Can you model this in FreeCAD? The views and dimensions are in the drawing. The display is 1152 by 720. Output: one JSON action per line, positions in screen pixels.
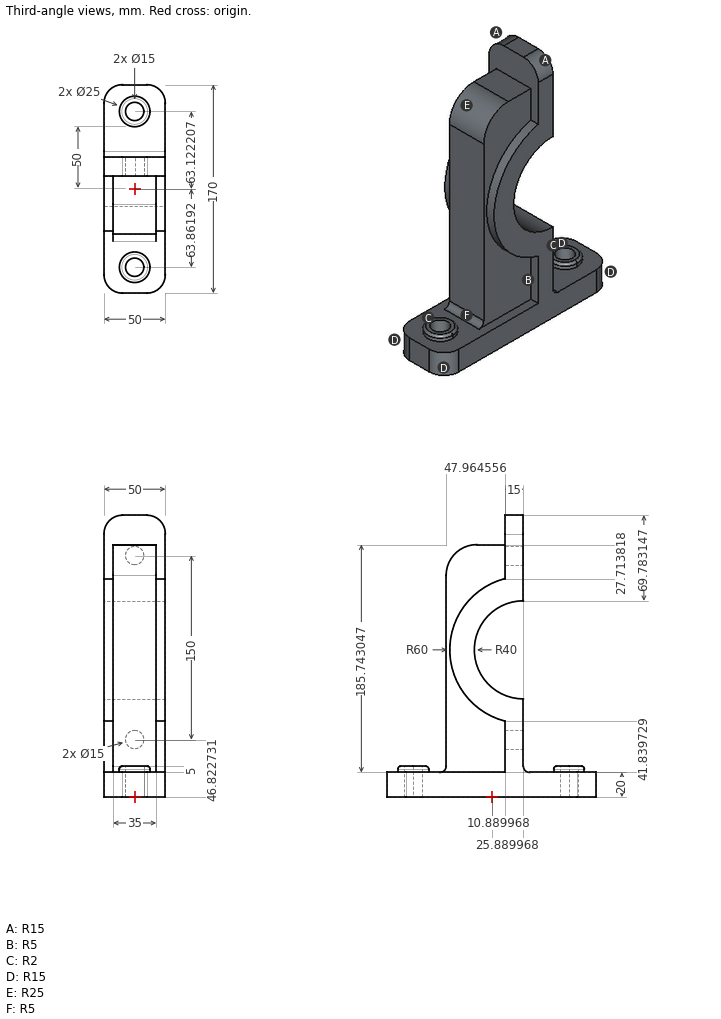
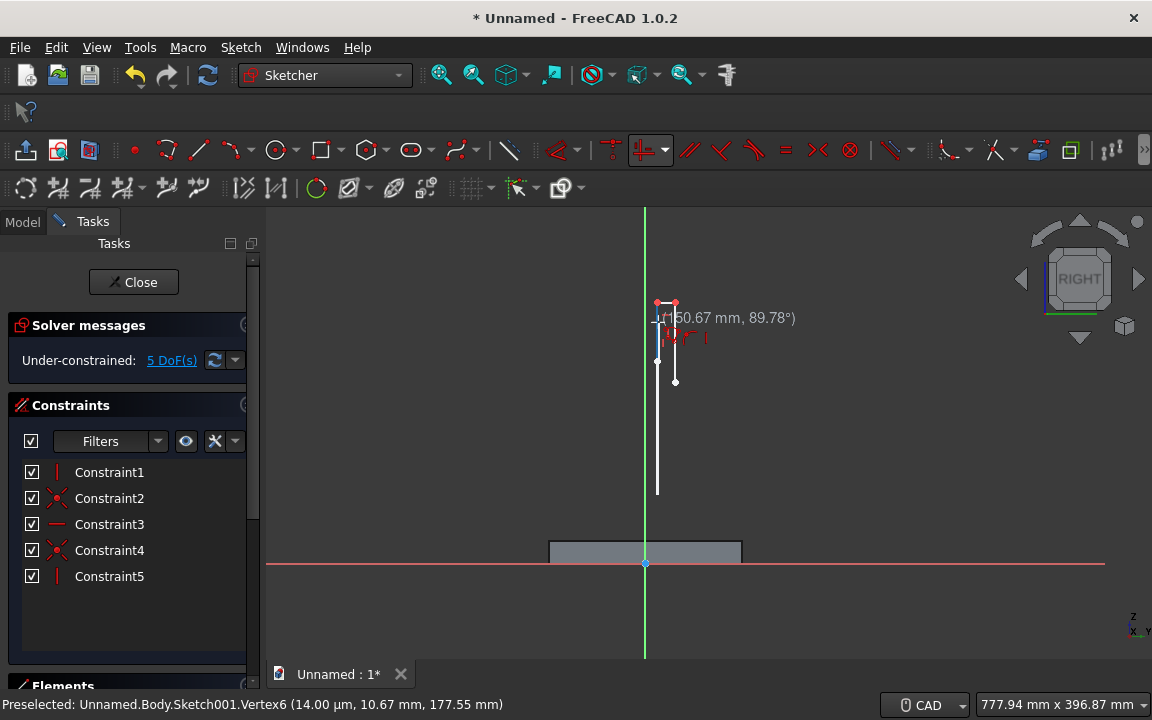
{"action": "scroll", "coordinate": [658, 541], "scroll_direction": "up", "scroll_amount": 2}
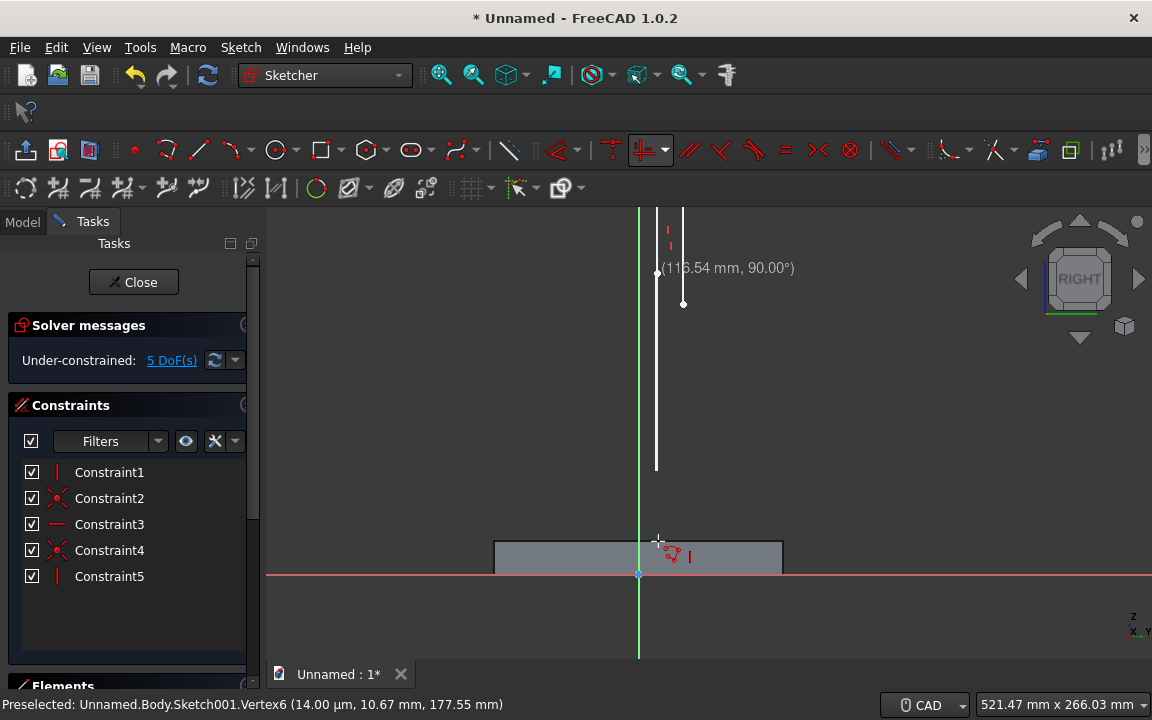
{"action": "left_click", "coordinate": [657, 541]}
{"action": "left_click", "coordinate": [683, 541]}
{"action": "left_click", "coordinate": [683, 439]}
{"action": "right_click", "coordinate": [683, 439]}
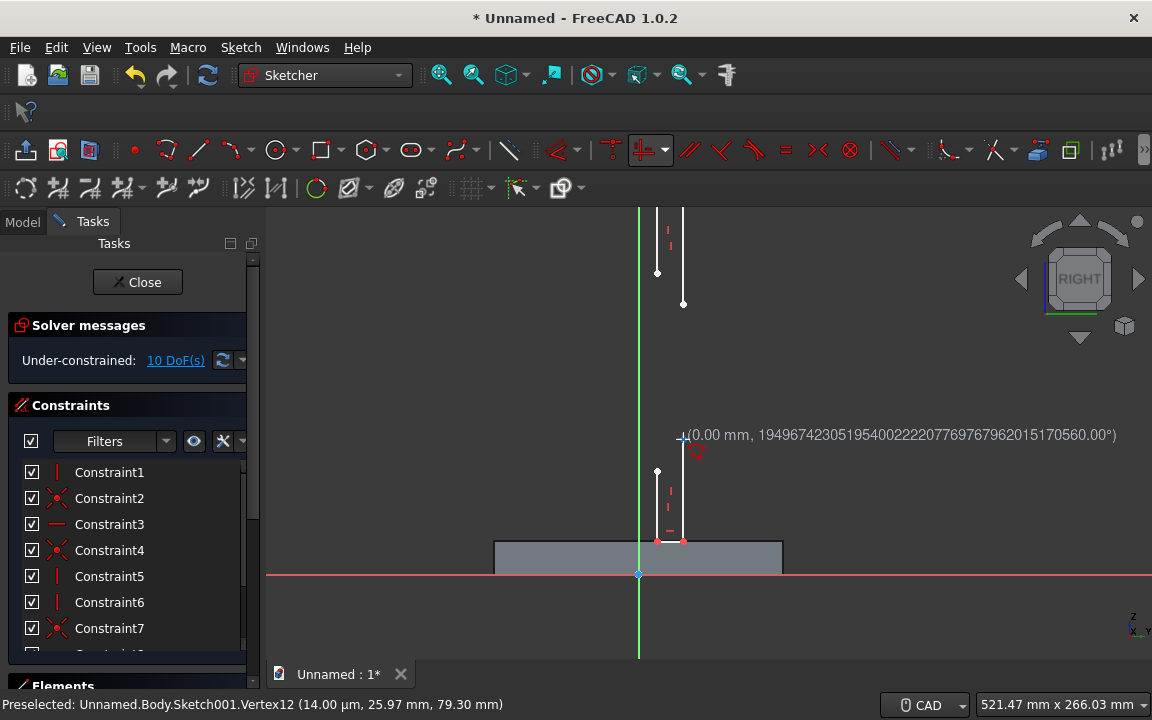
{"action": "key", "text": "g 3 a"}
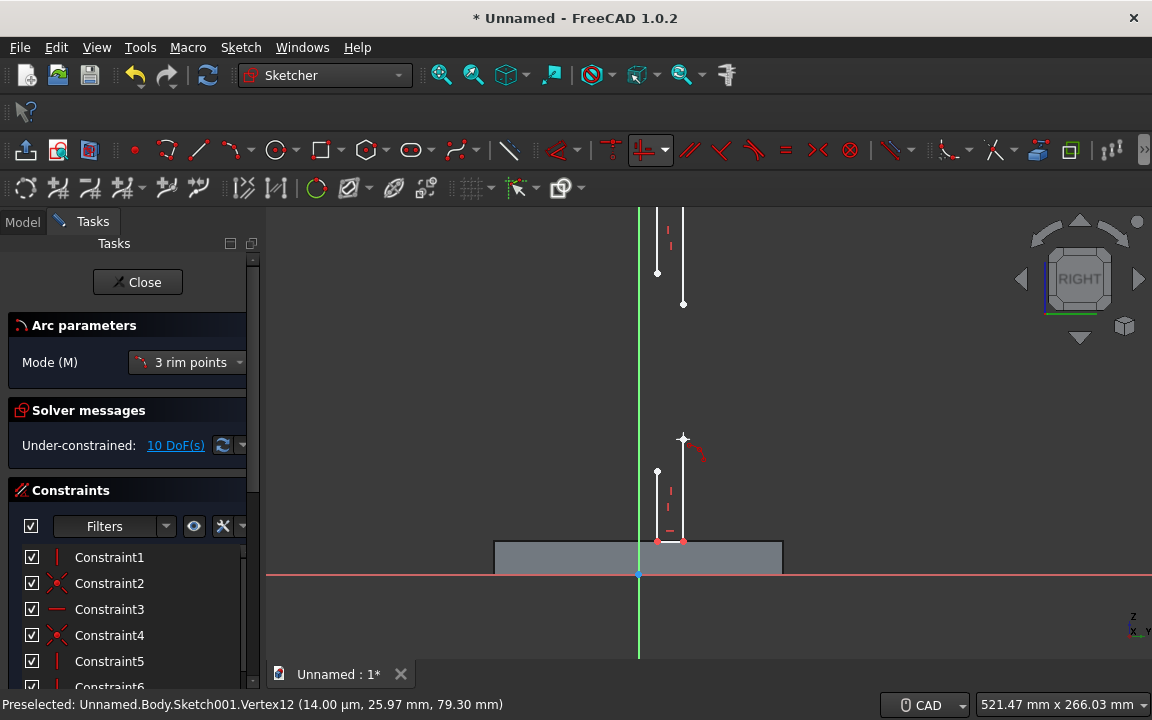
{"action": "left_click", "coordinate": [657, 273]}
{"action": "left_click", "coordinate": [657, 471]}
{"action": "left_click", "coordinate": [581, 371]}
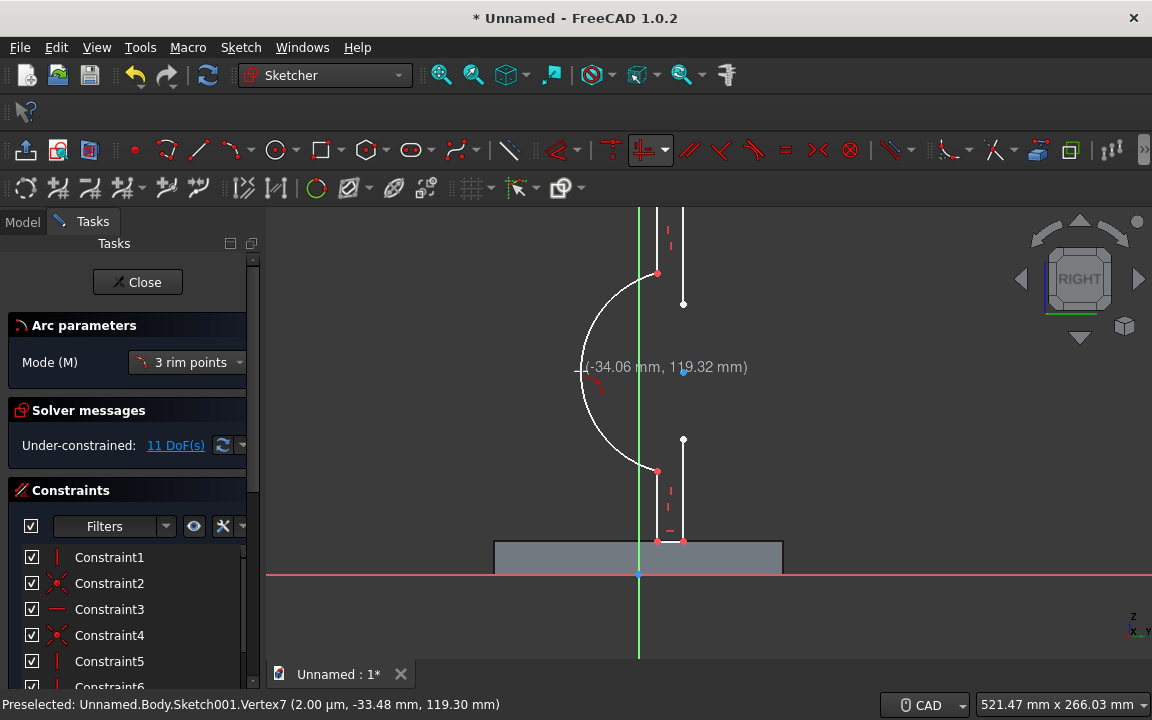
{"action": "left_click", "coordinate": [683, 440]}
{"action": "left_click", "coordinate": [683, 305]}
{"action": "left_click", "coordinate": [615, 371]}
{"action": "key", "text": "Escape"}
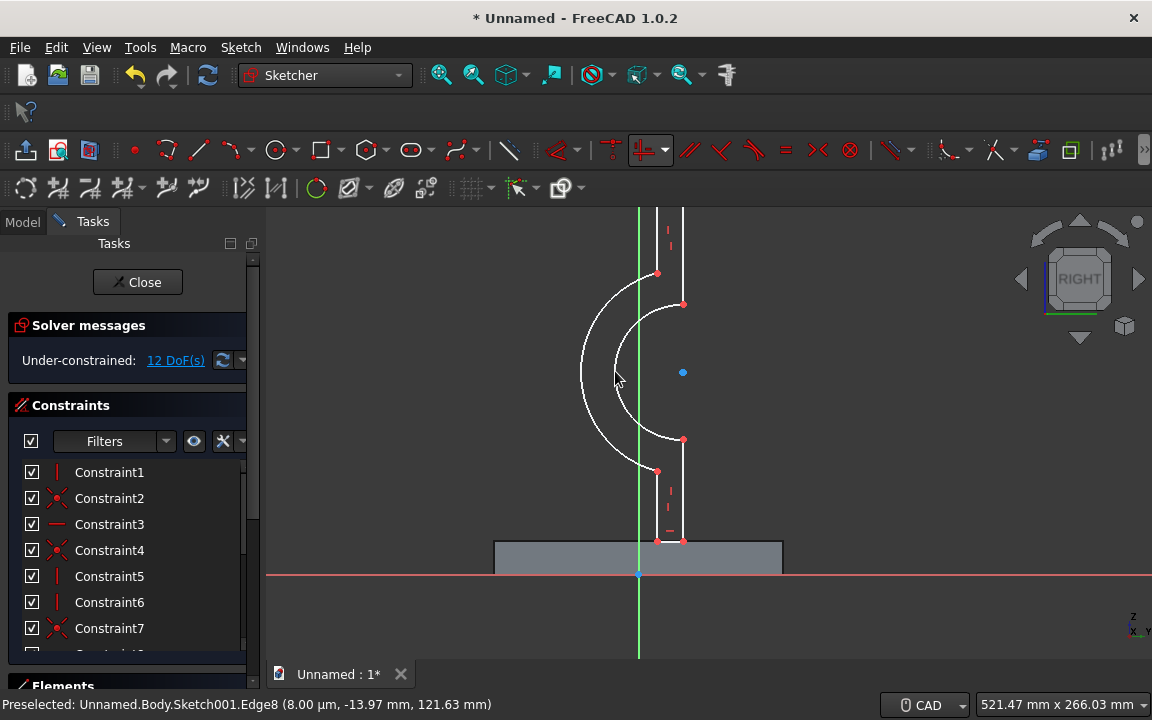
{"action": "left_click", "coordinate": [595, 321]}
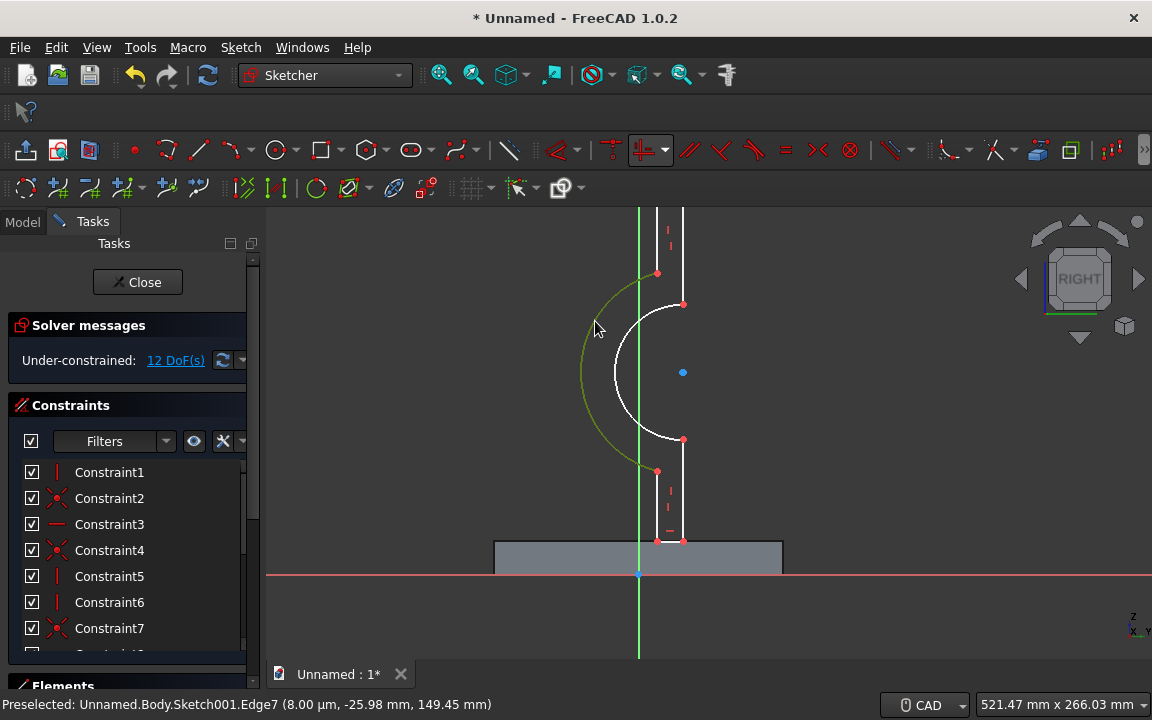
{"action": "scroll", "coordinate": [628, 332], "scroll_direction": "up", "scroll_amount": 2}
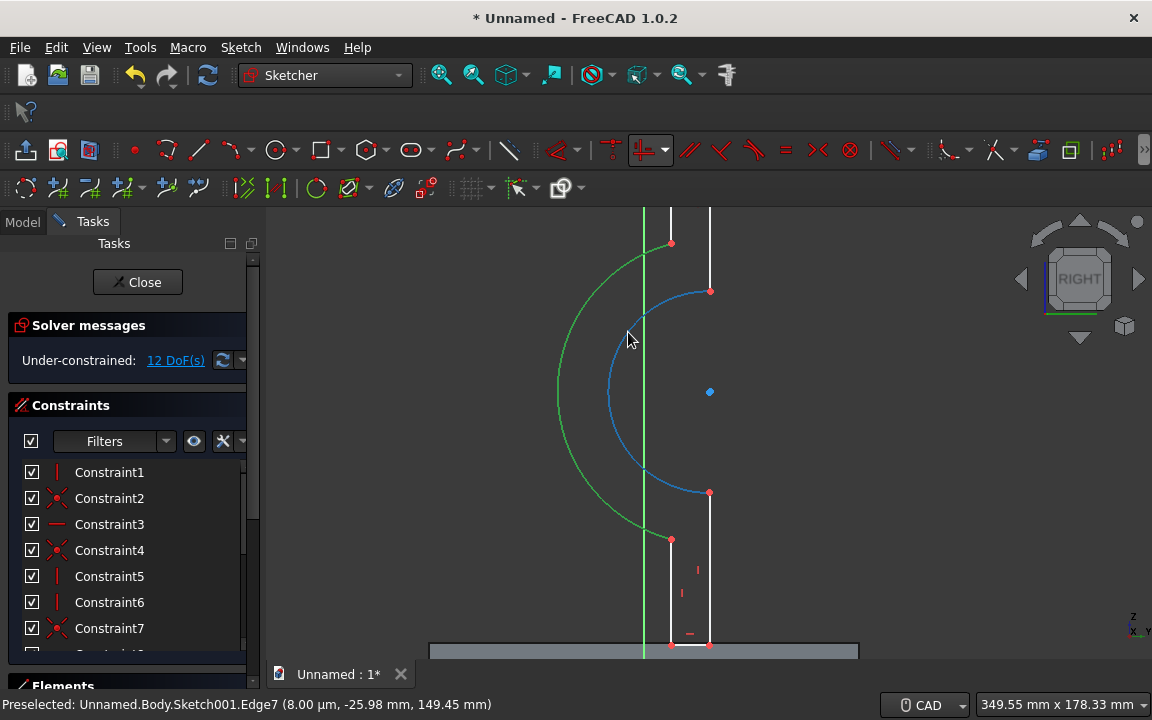
{"action": "left_click", "coordinate": [628, 333]}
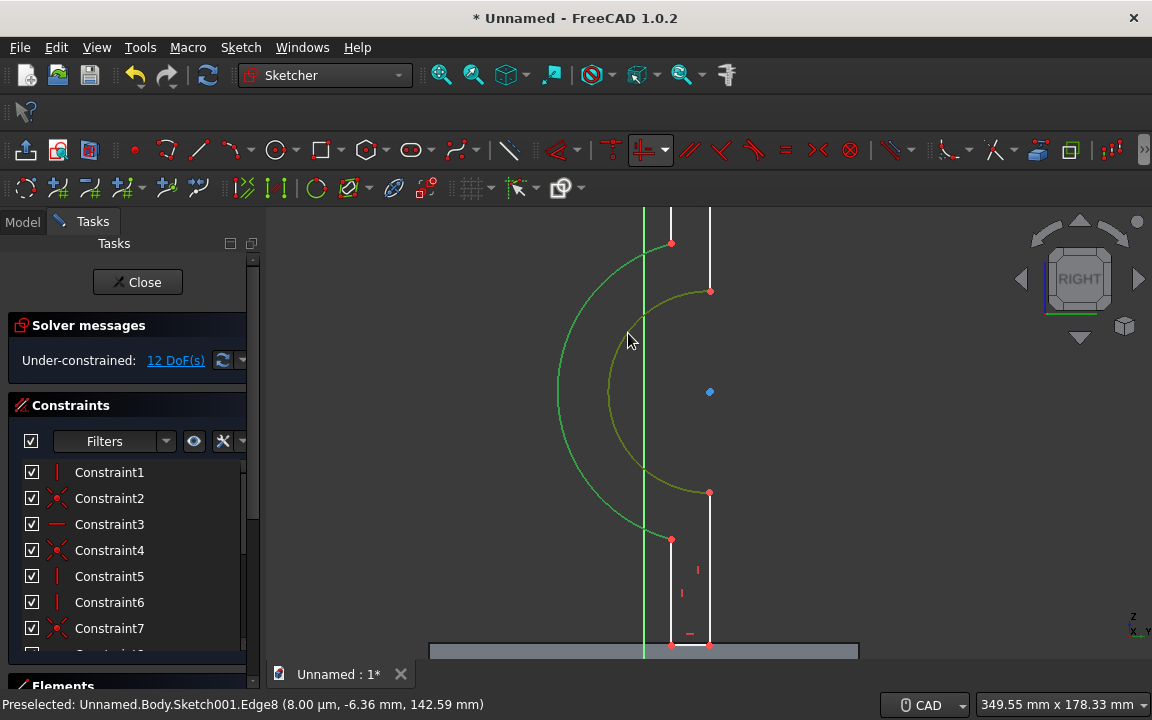
{"action": "key", "text": "c"}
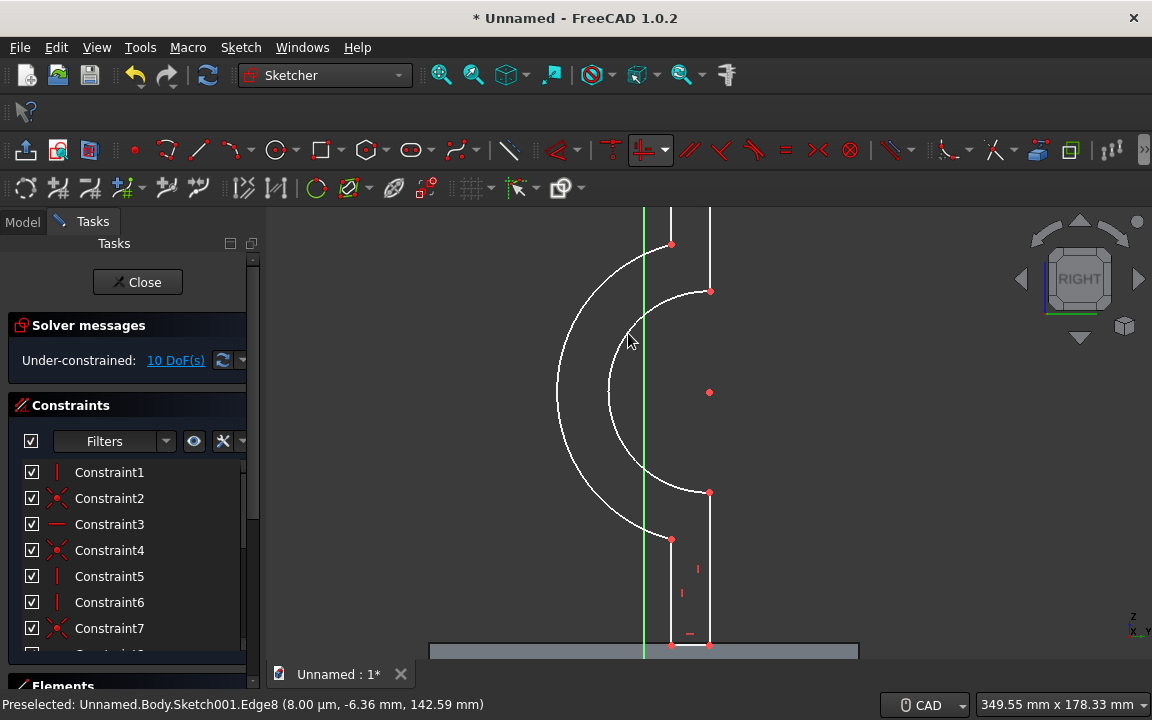
{"action": "left_click", "coordinate": [578, 316]}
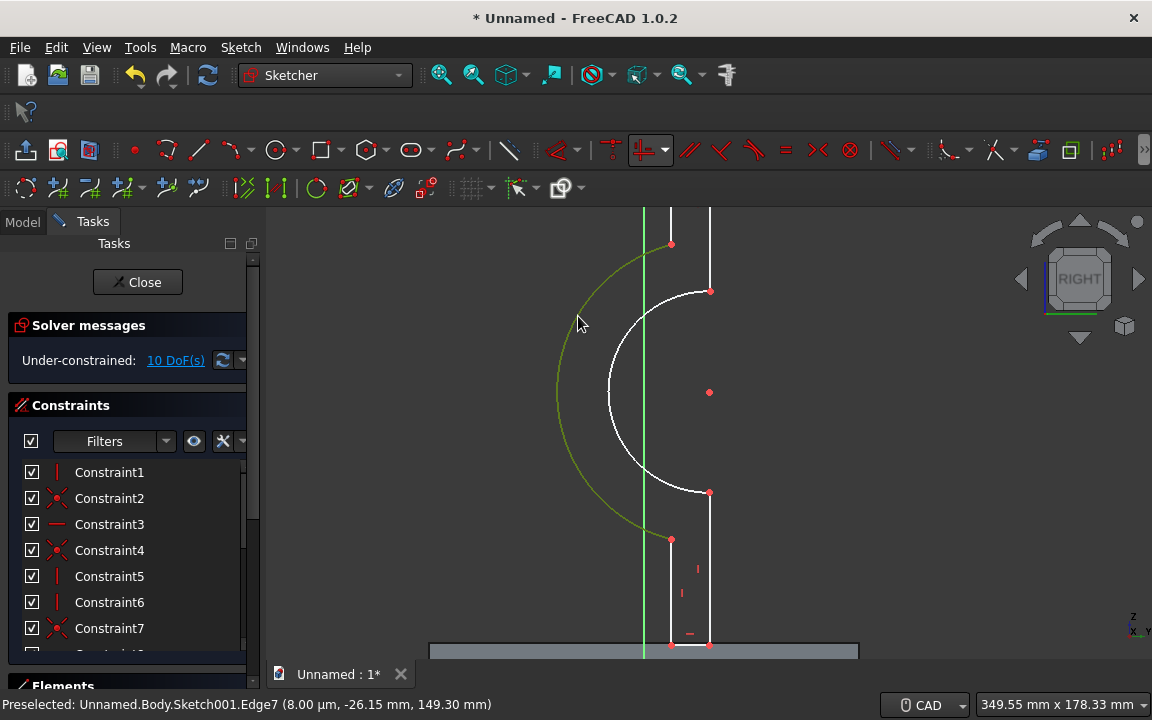
{"action": "key", "text": "k r"}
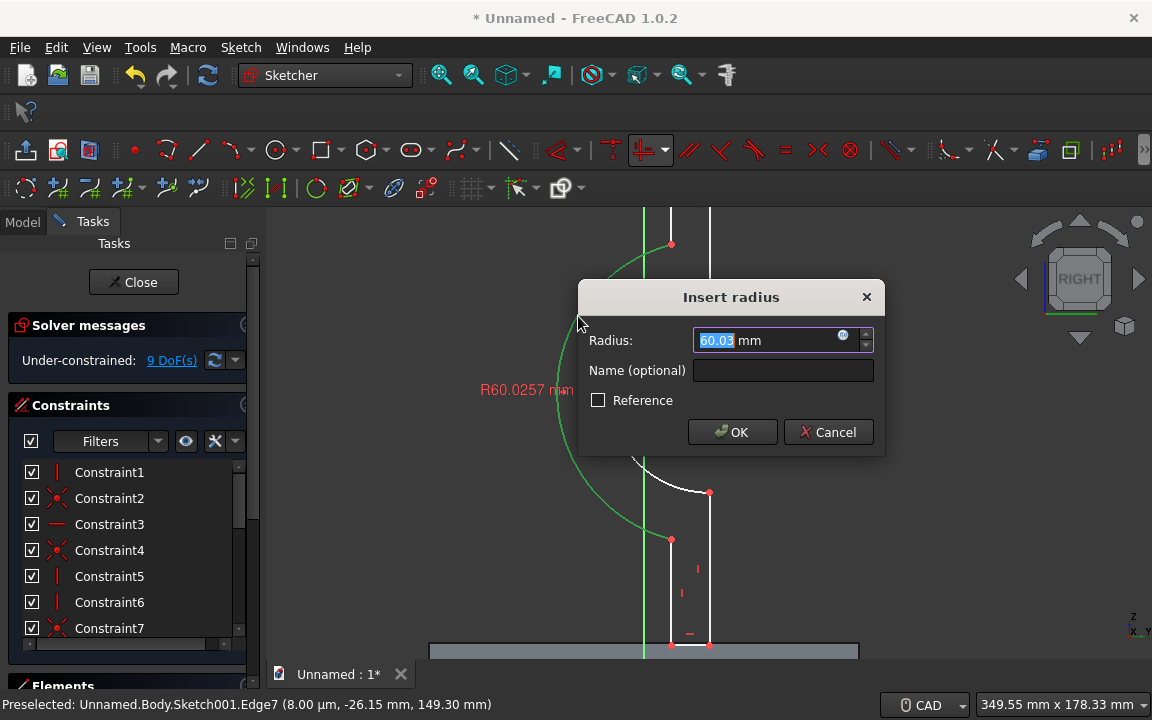
{"action": "type", "text": "60"}
{"action": "key", "text": "Return"}